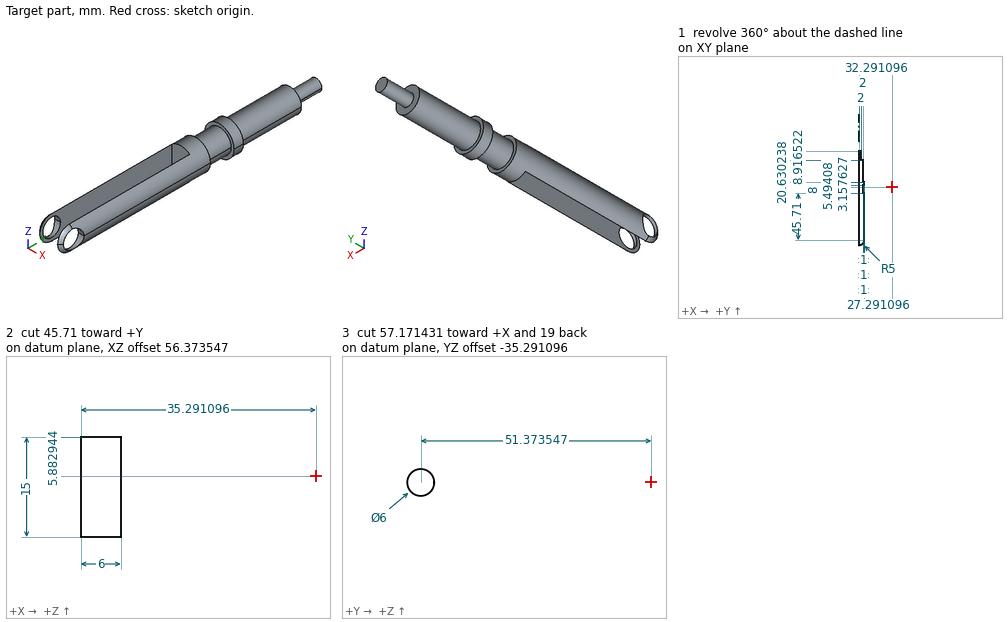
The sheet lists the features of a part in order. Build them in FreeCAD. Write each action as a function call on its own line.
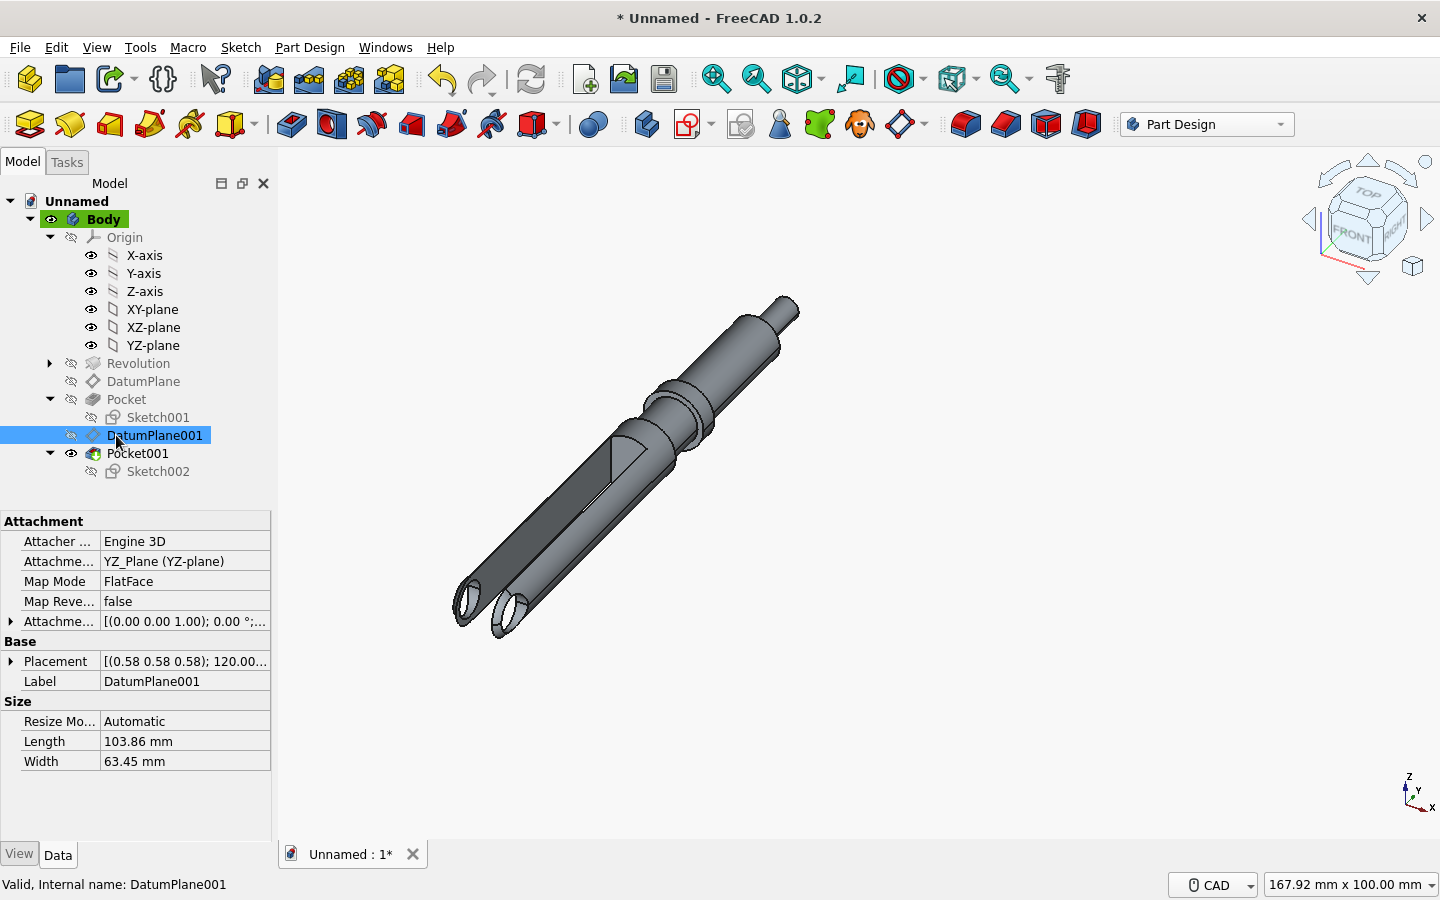
key(0)